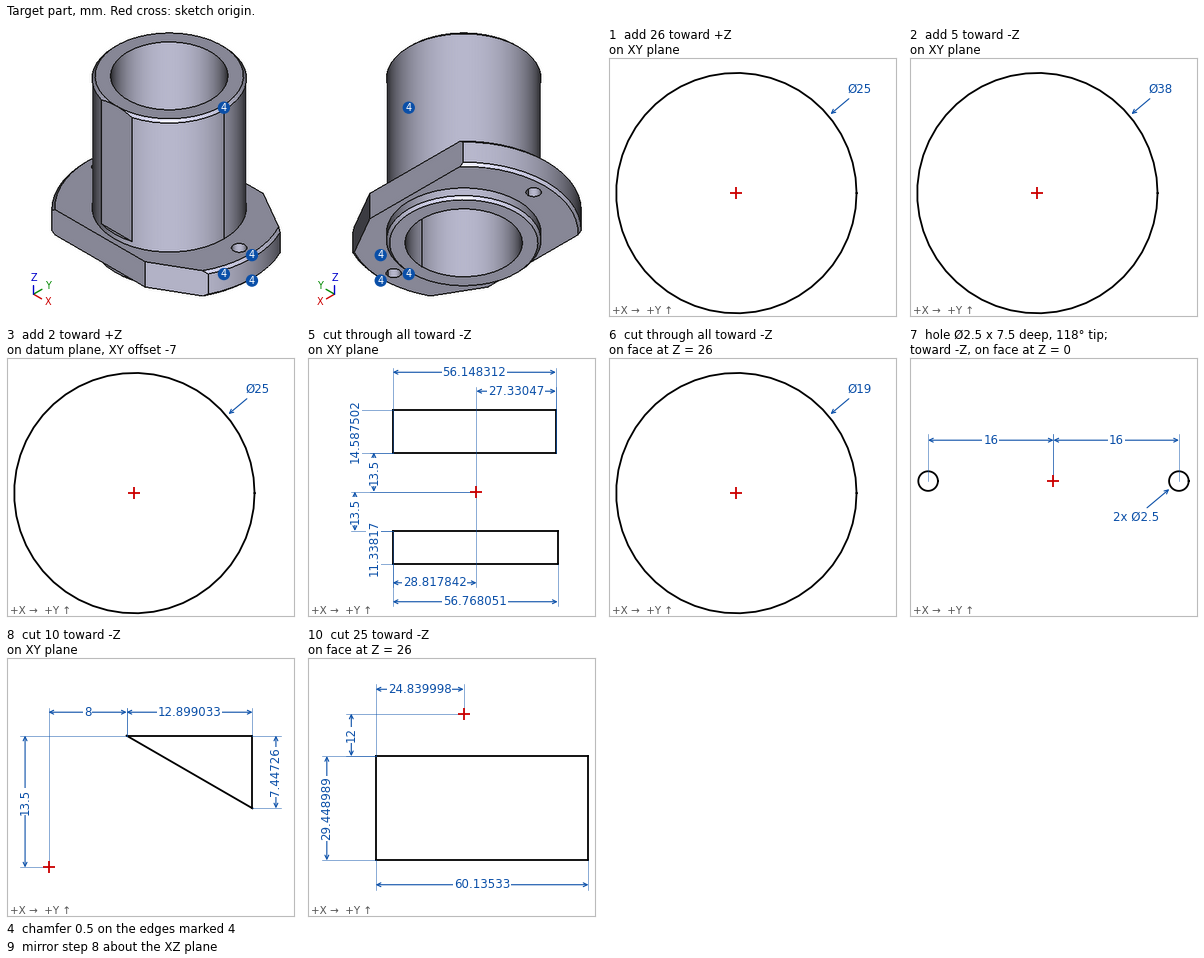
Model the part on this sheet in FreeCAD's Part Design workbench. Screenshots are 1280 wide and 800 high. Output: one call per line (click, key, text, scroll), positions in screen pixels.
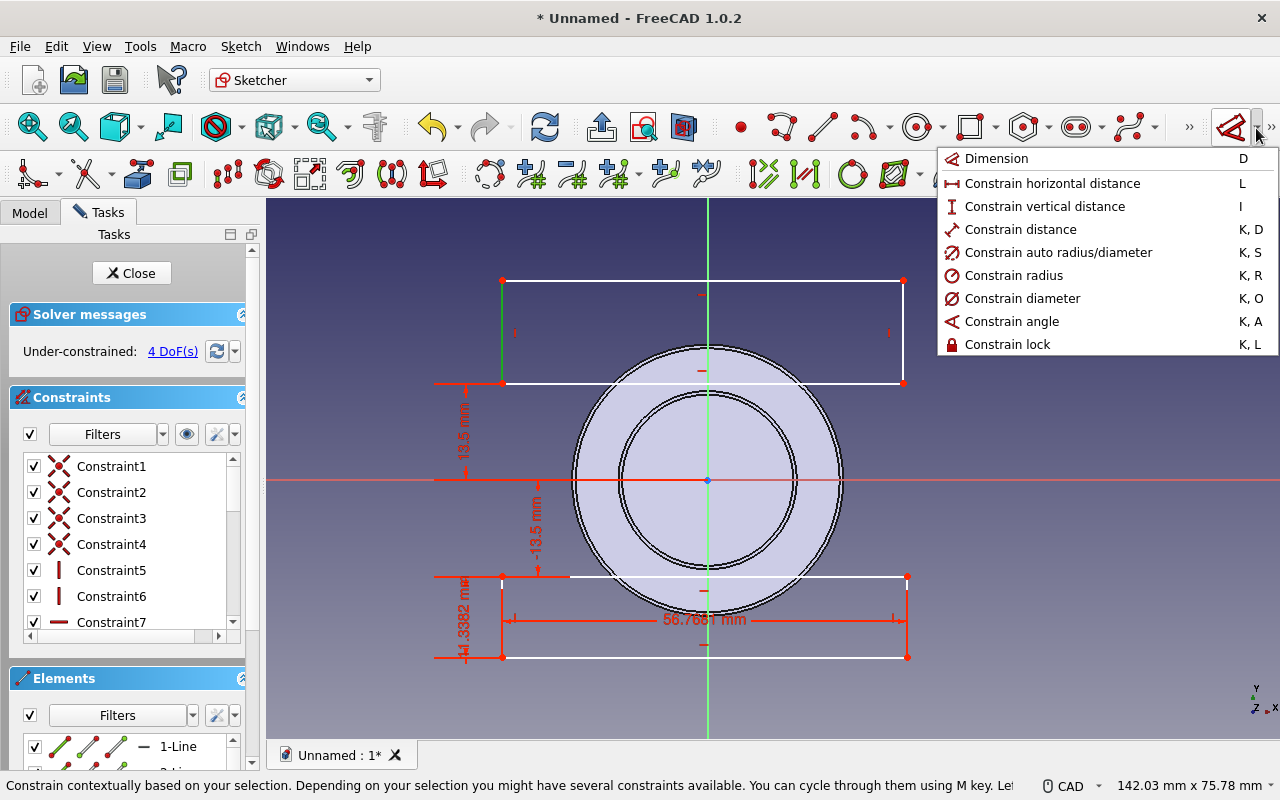
click(1108, 206)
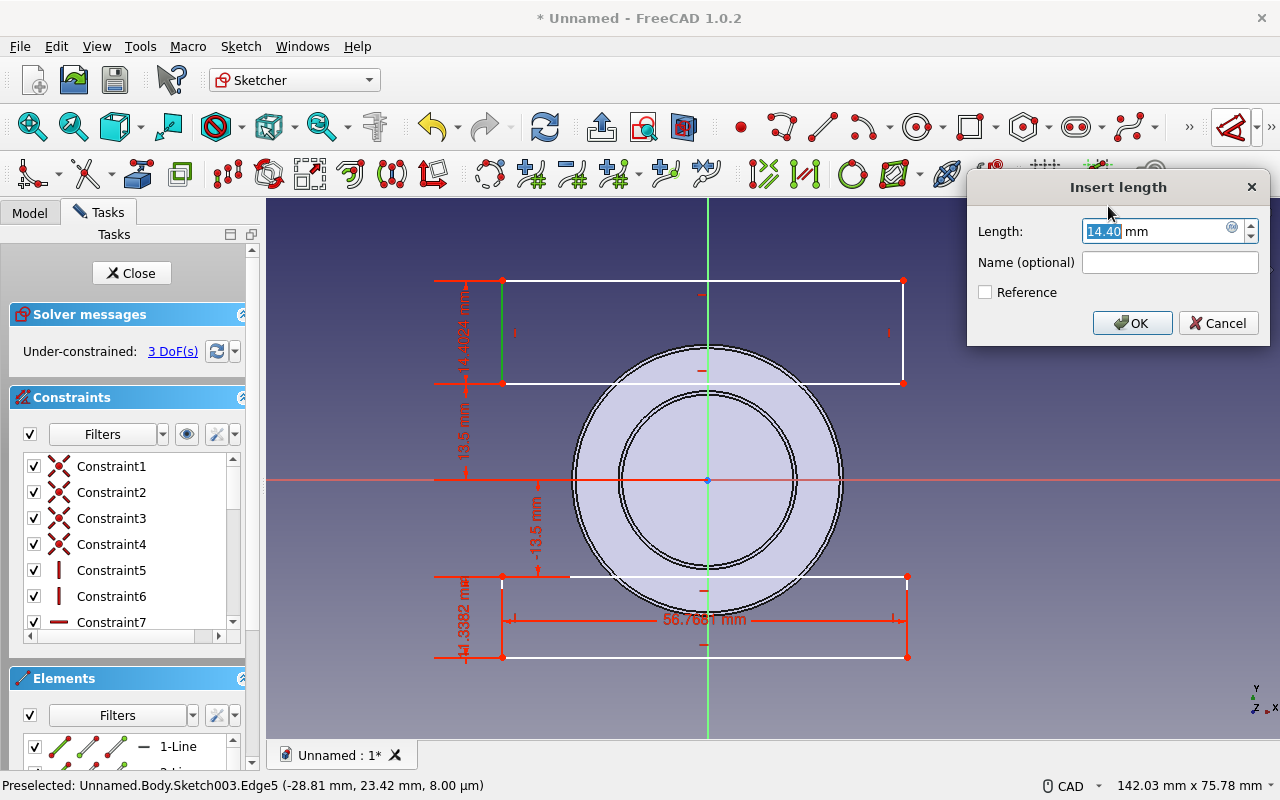
text(14.587502)
key(Return)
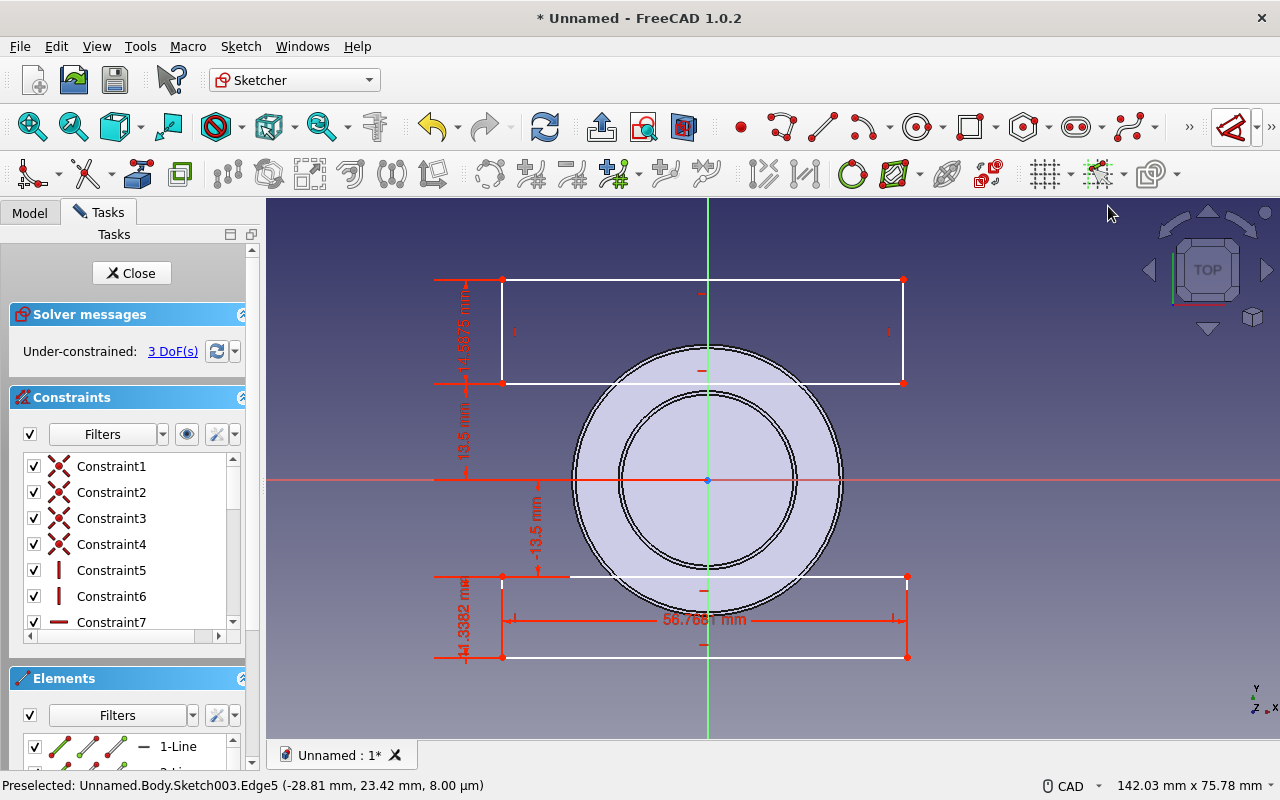
click(622, 384)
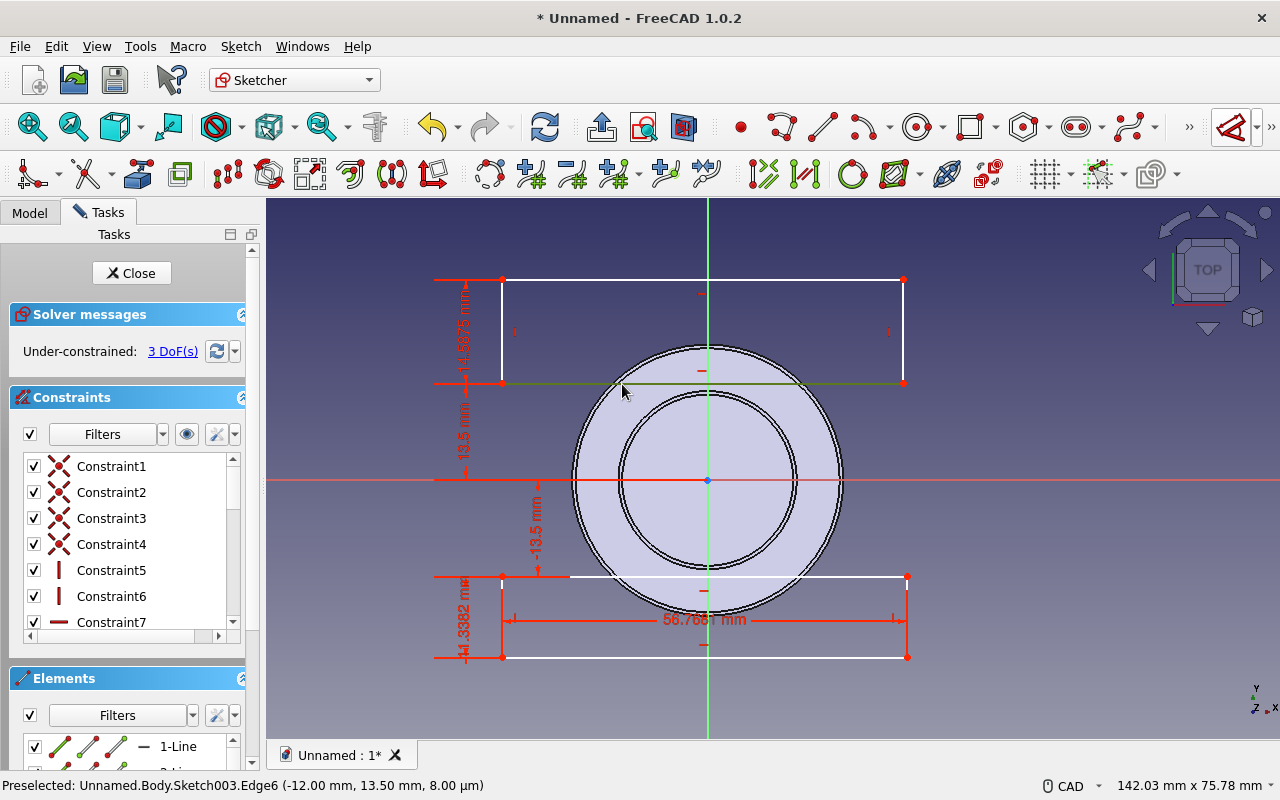
key(l)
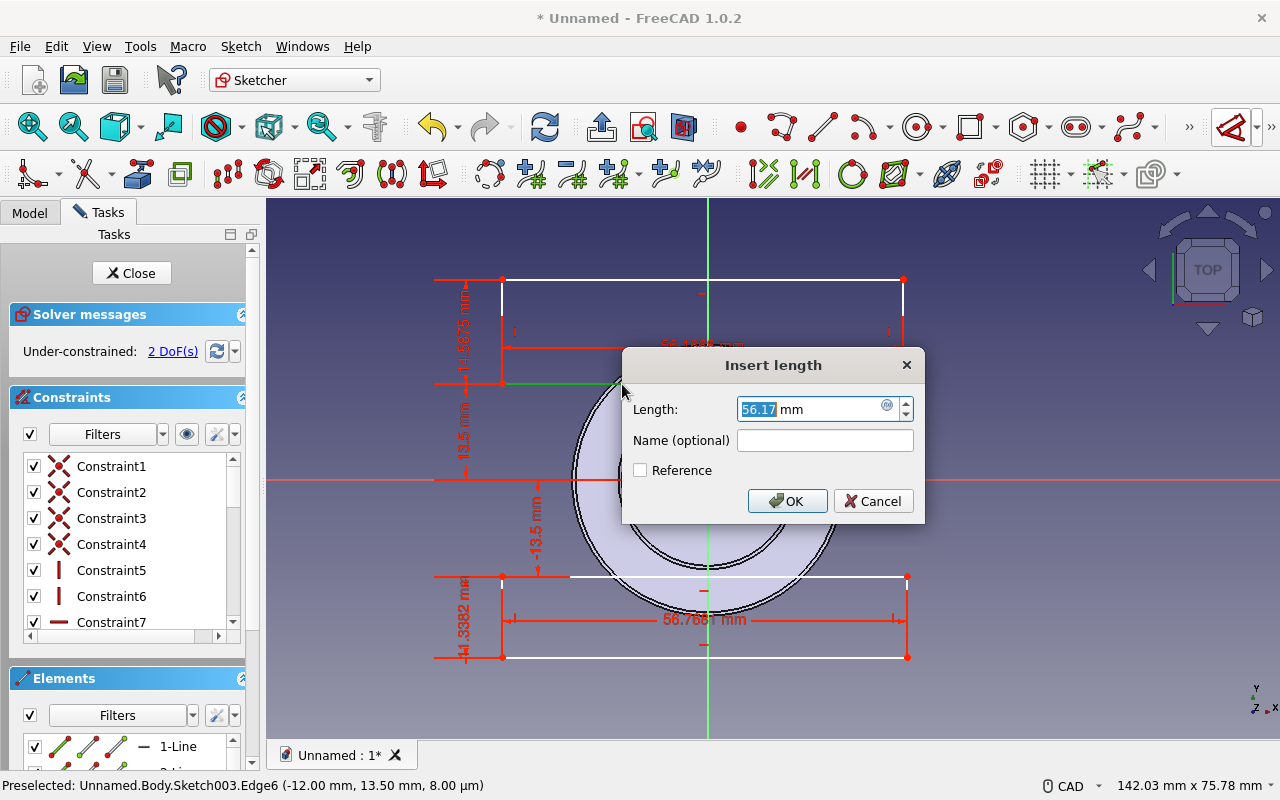
text(56.148312)
key(Return)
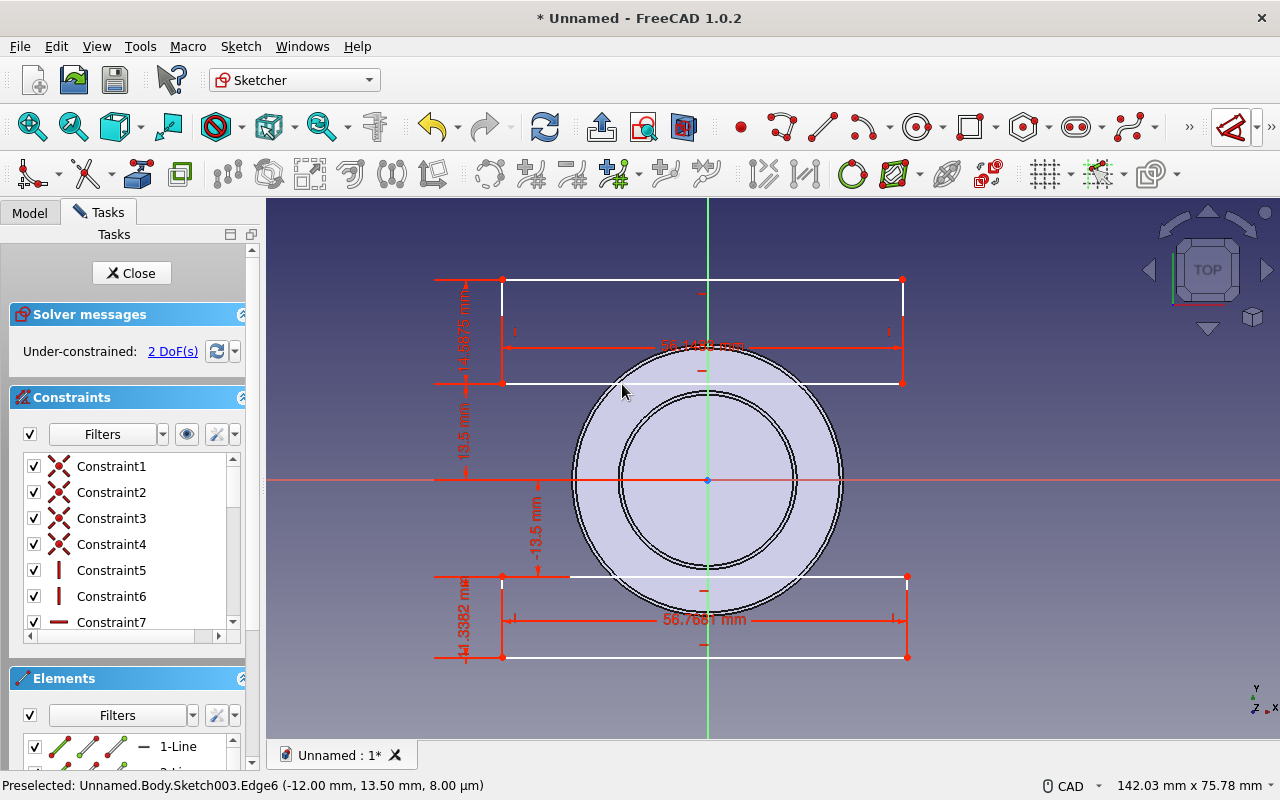
click(903, 384)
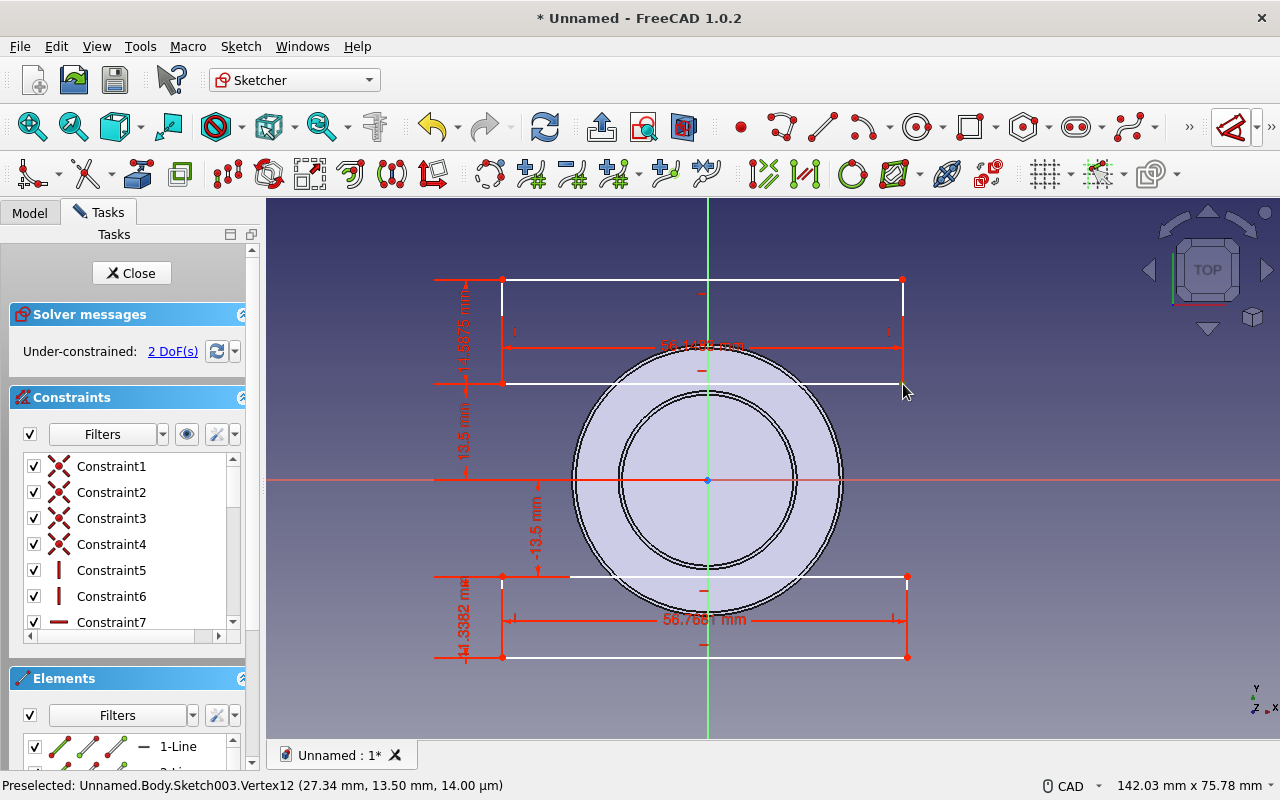
click(1256, 128)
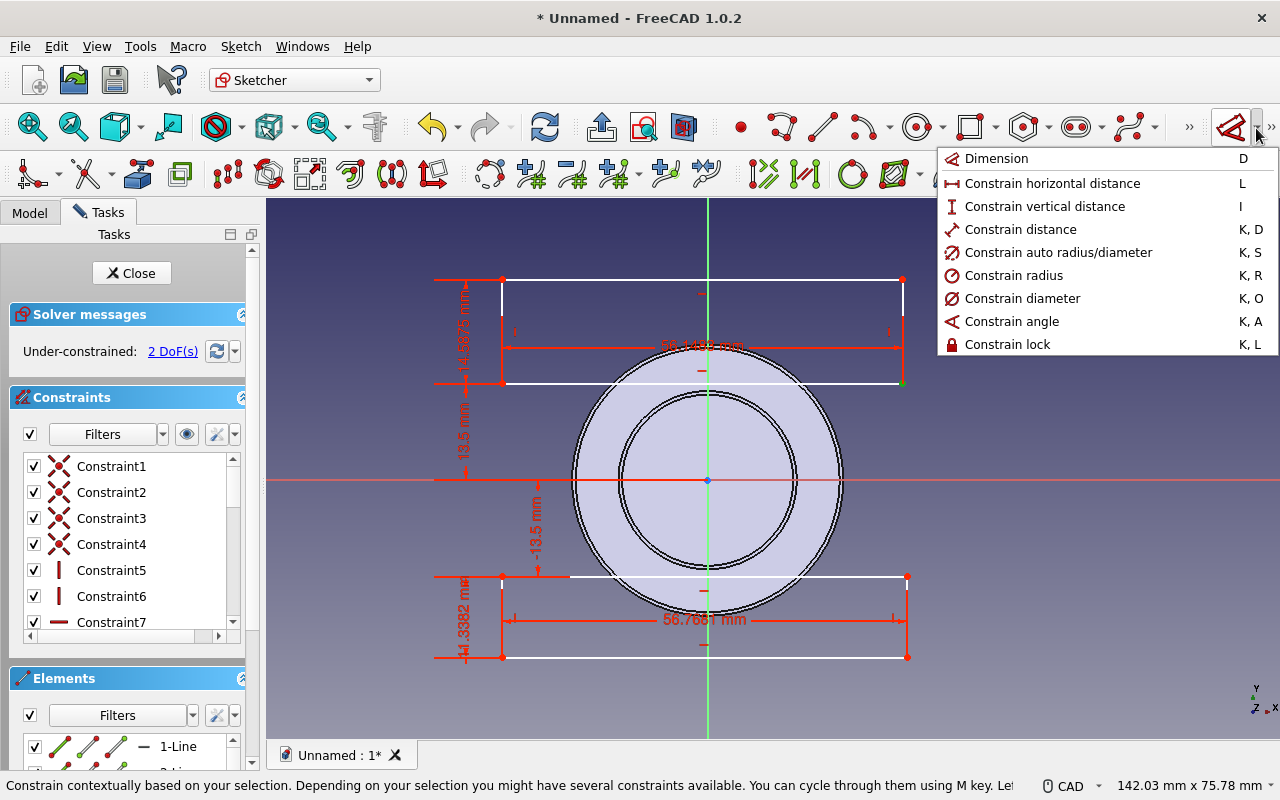
click(1108, 184)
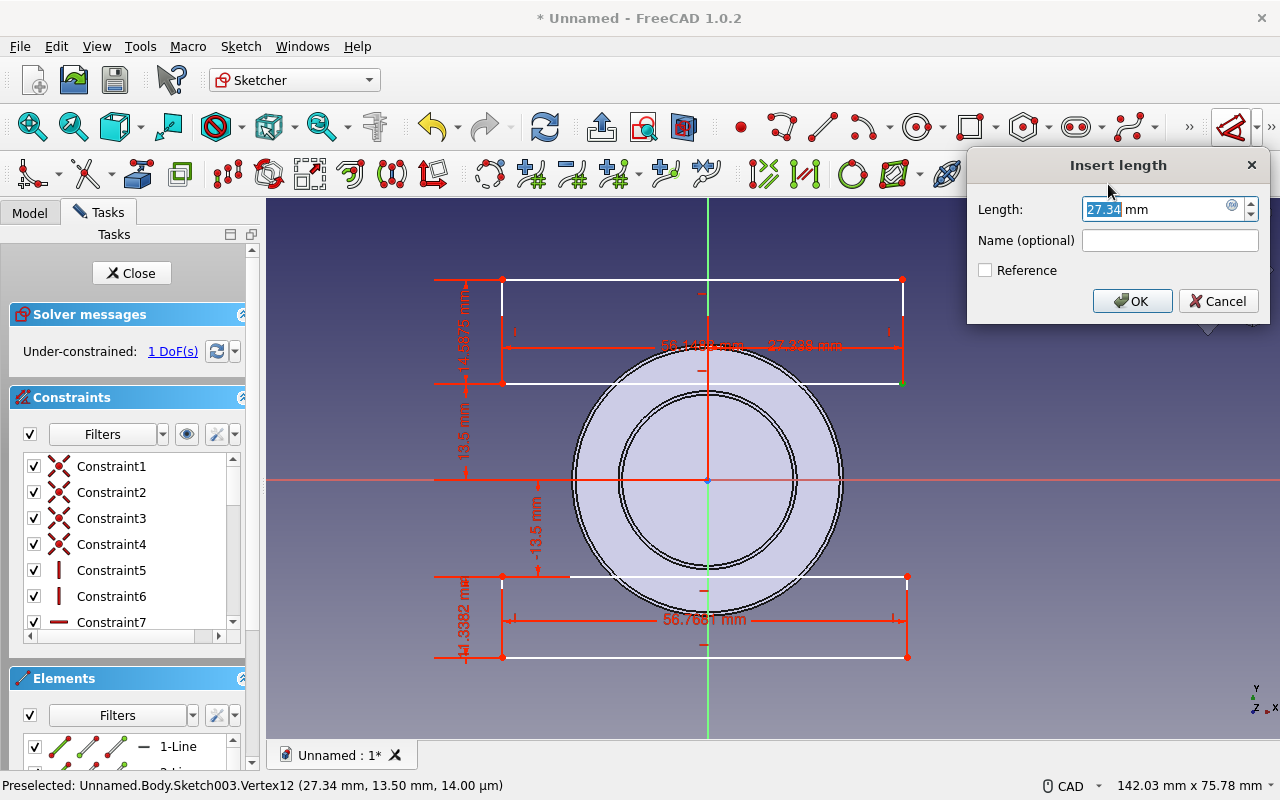
text(27.33047)
key(Return)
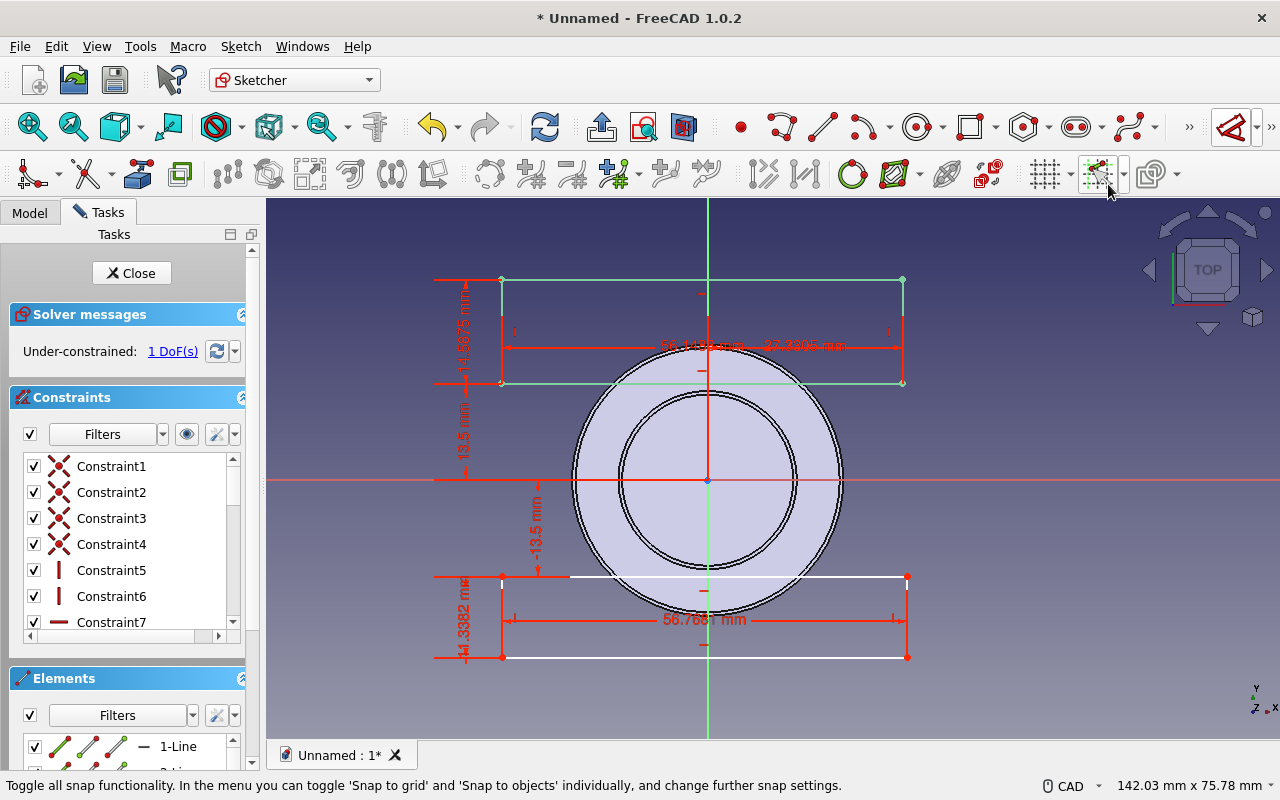
click(502, 577)